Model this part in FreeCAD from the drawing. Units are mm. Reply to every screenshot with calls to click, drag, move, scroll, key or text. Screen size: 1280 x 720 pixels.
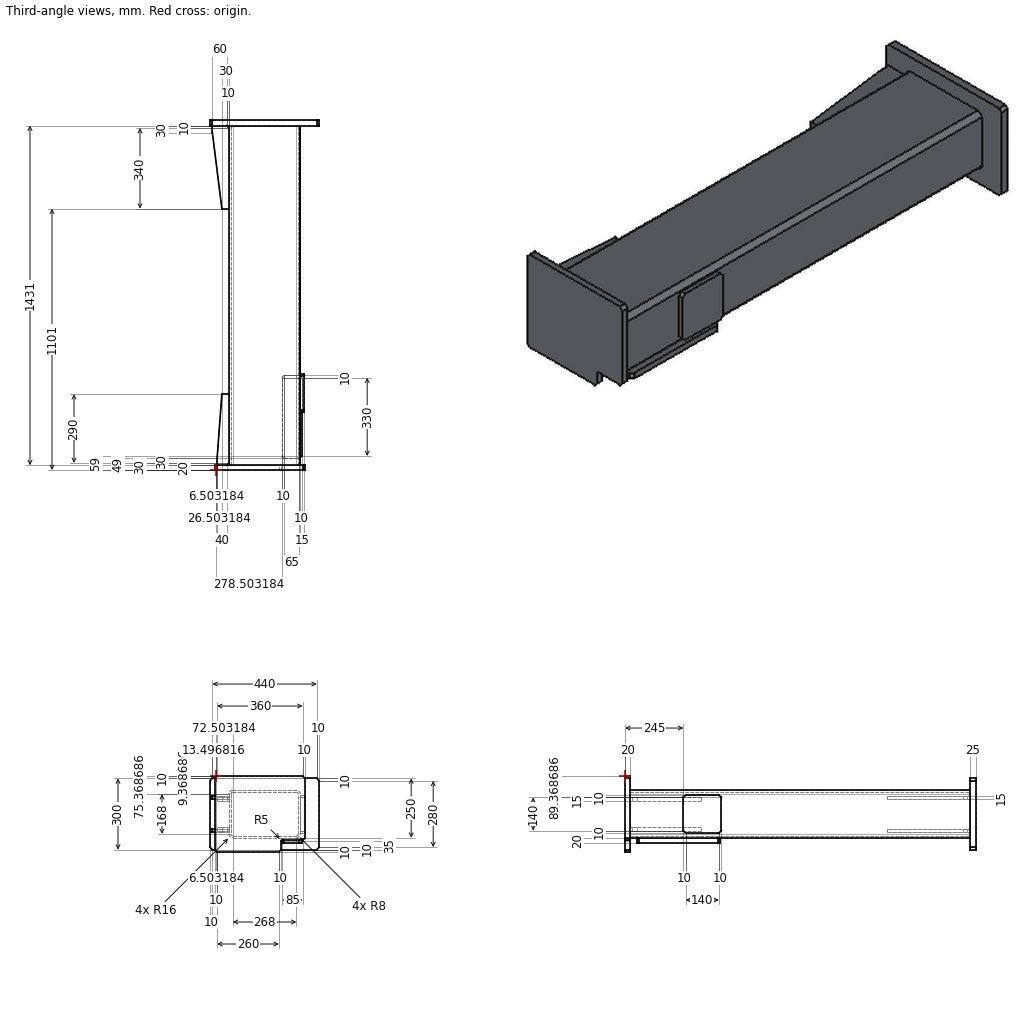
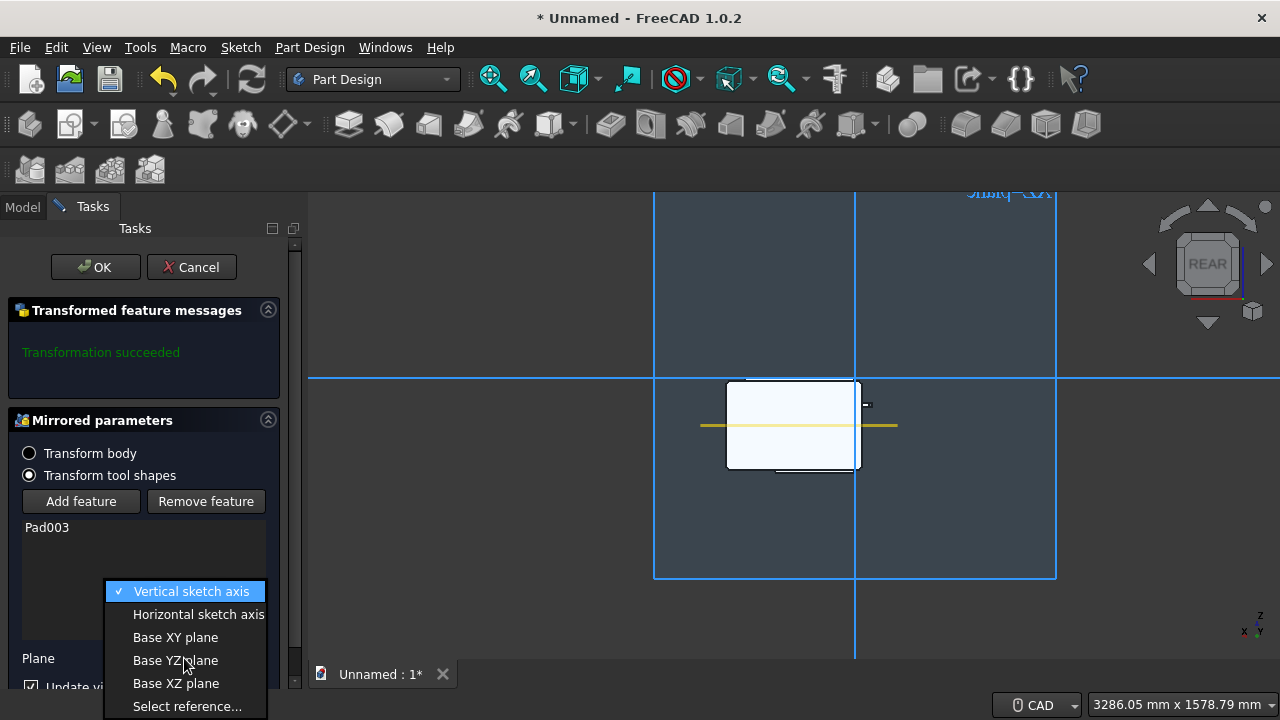
click(184, 706)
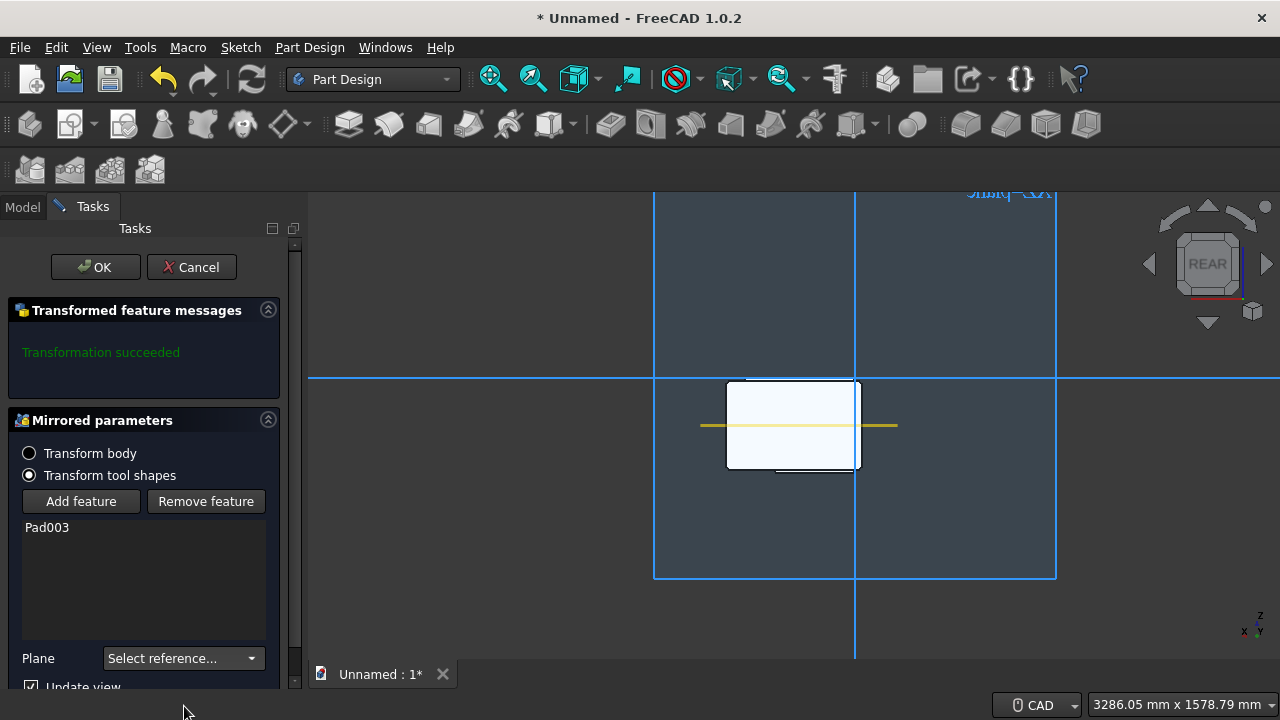
click(23, 206)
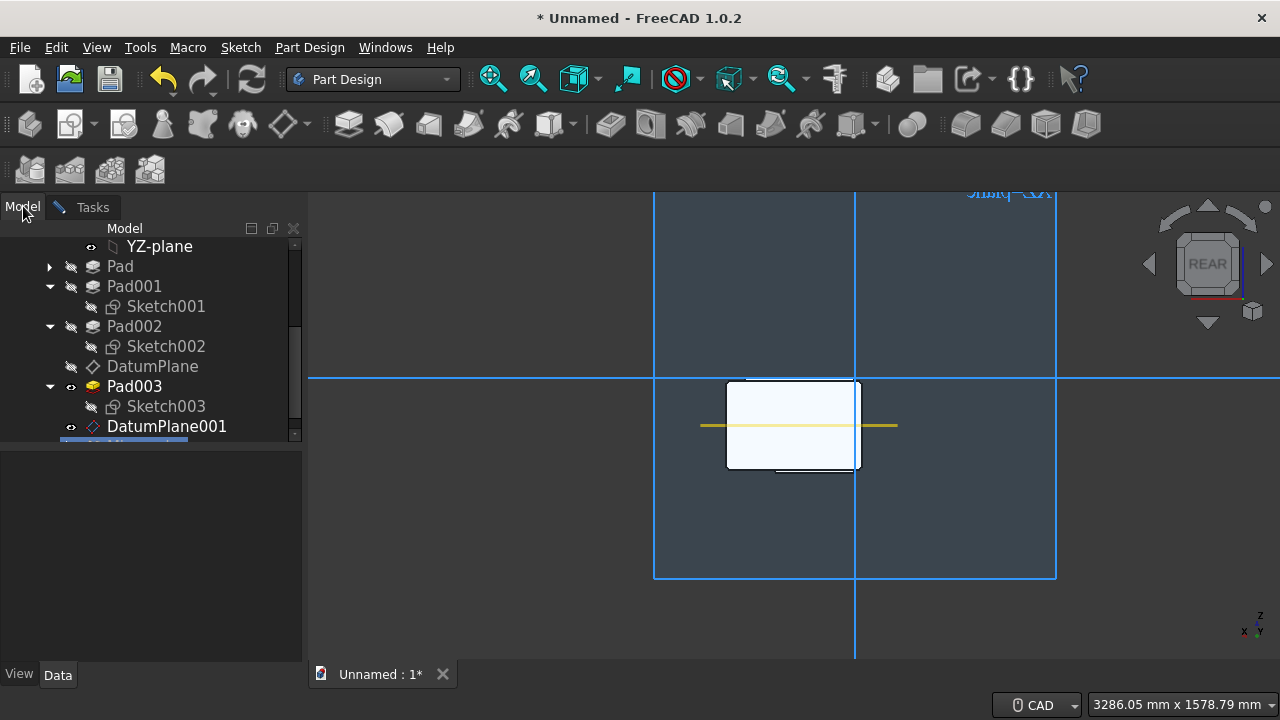
click(116, 427)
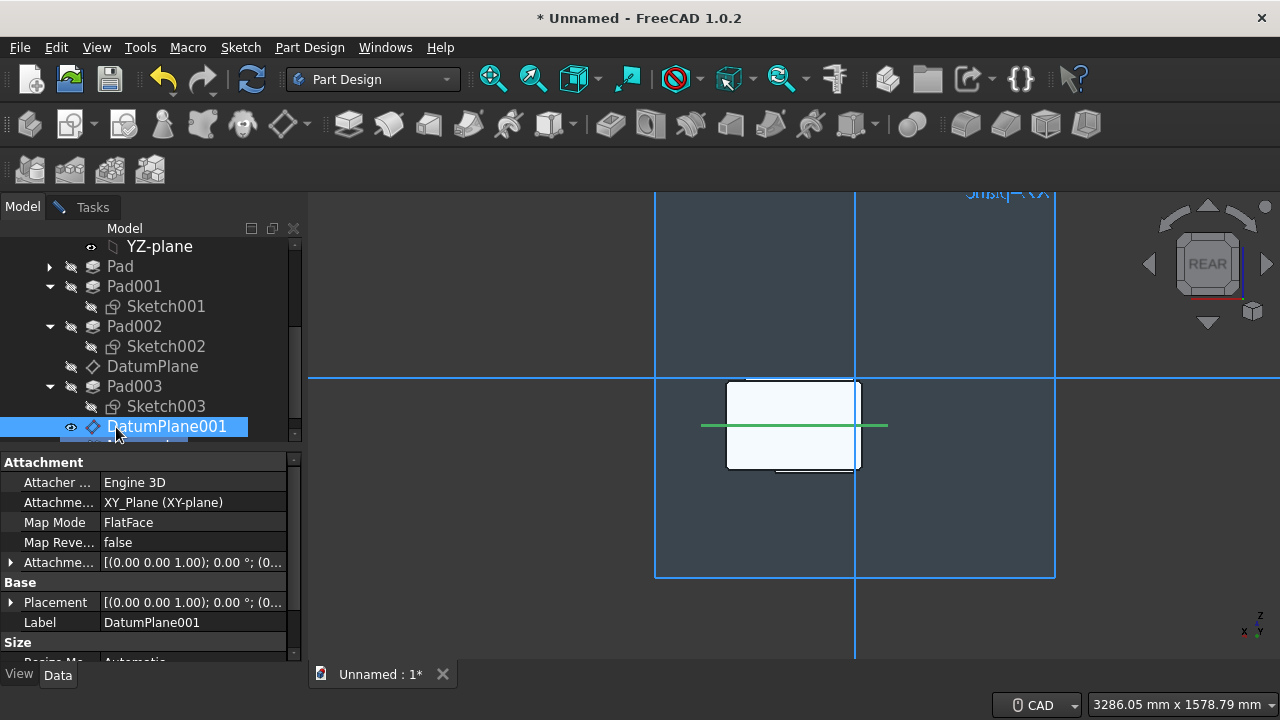
click(84, 206)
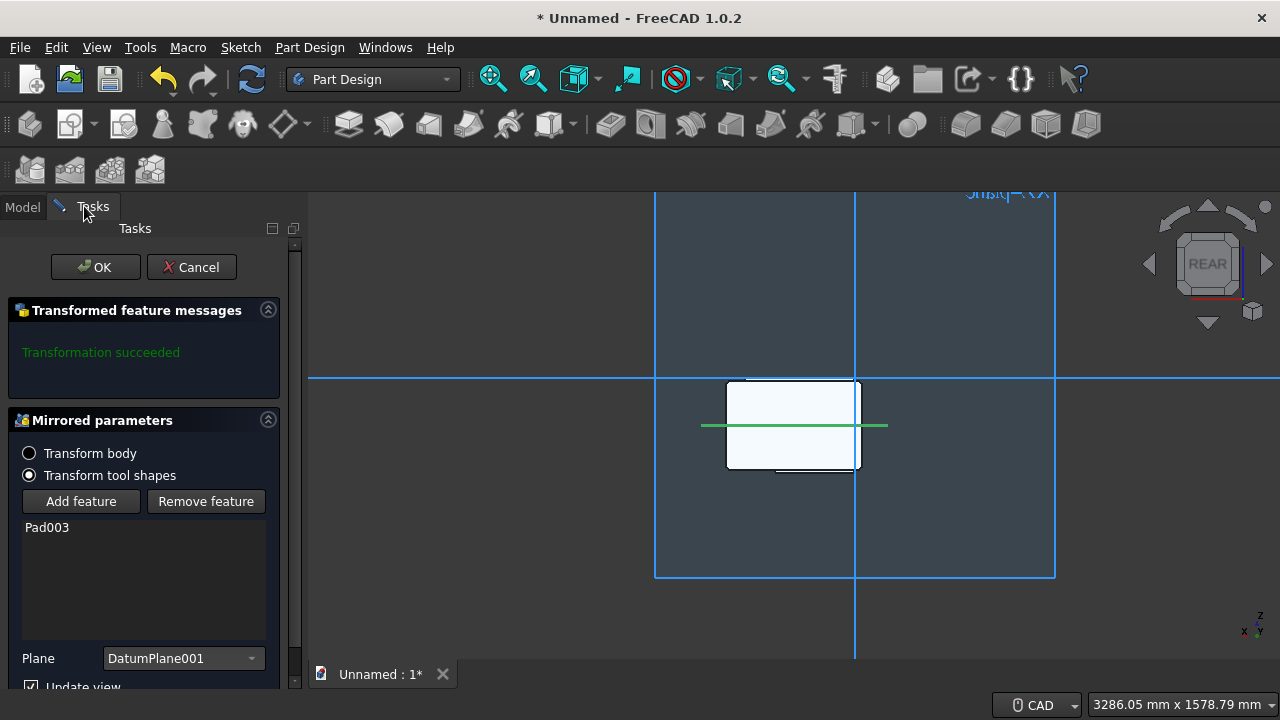
click(96, 267)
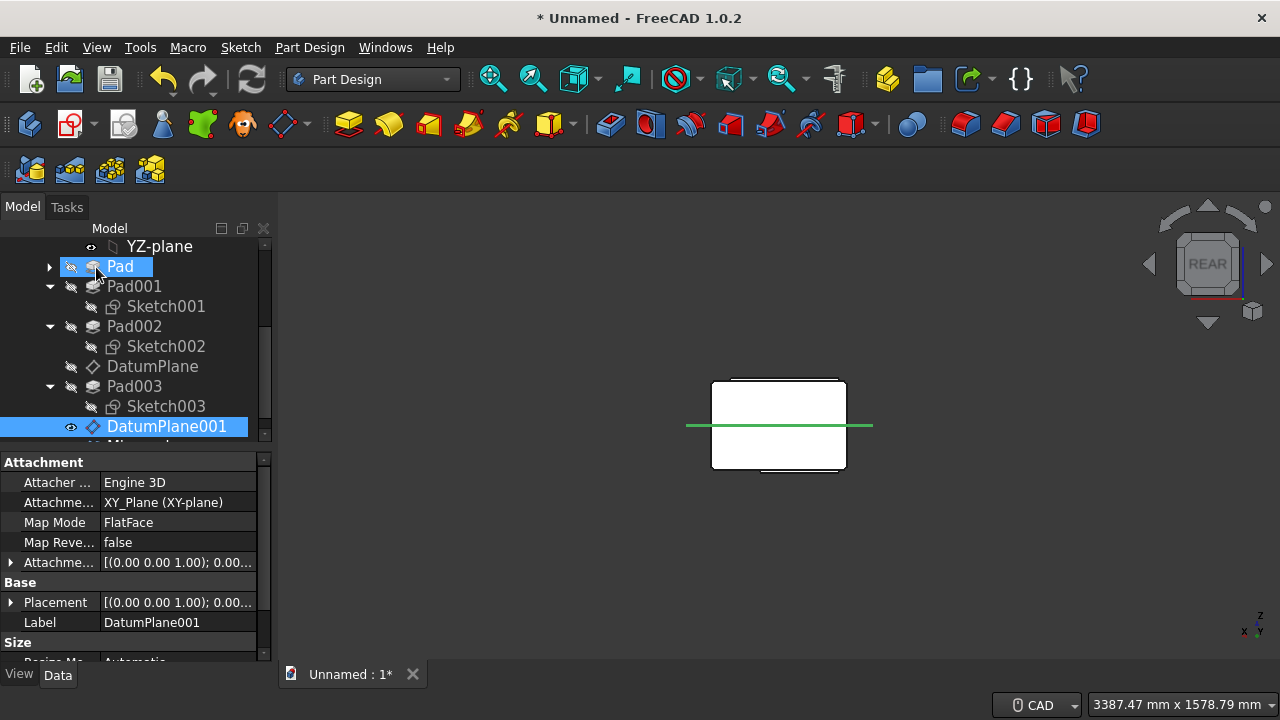
click(116, 427)
key(space)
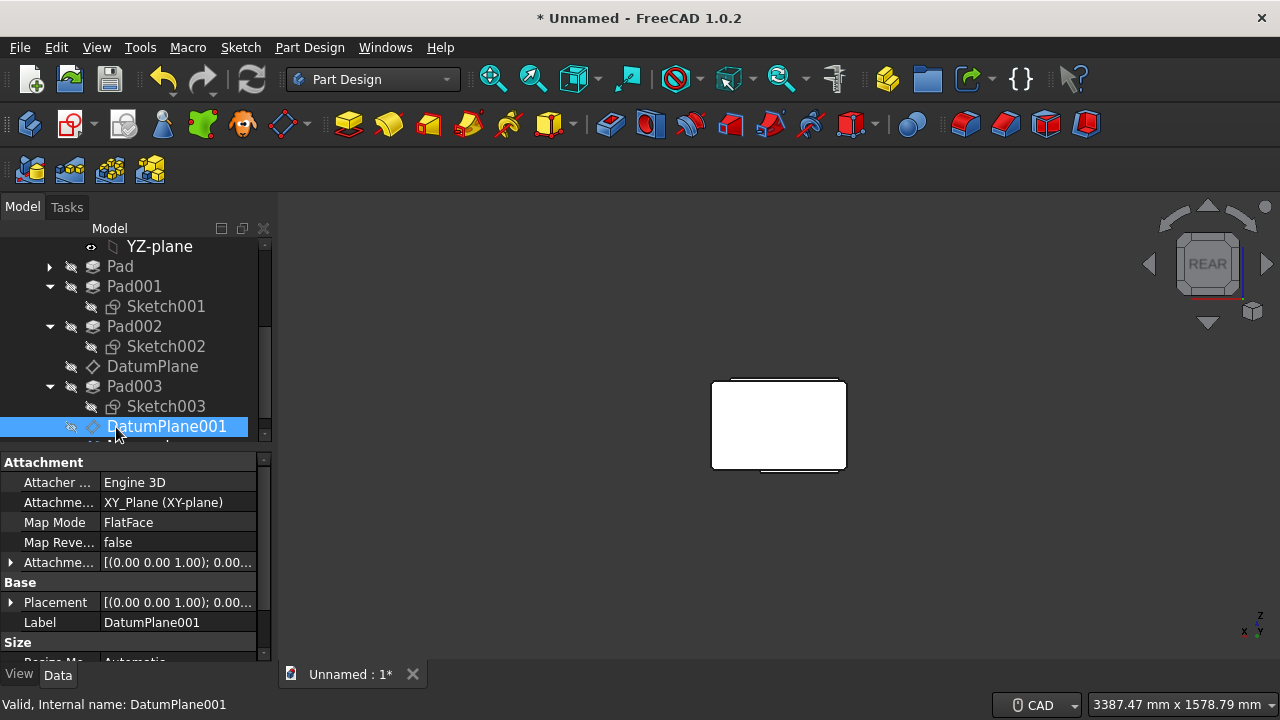
click(494, 80)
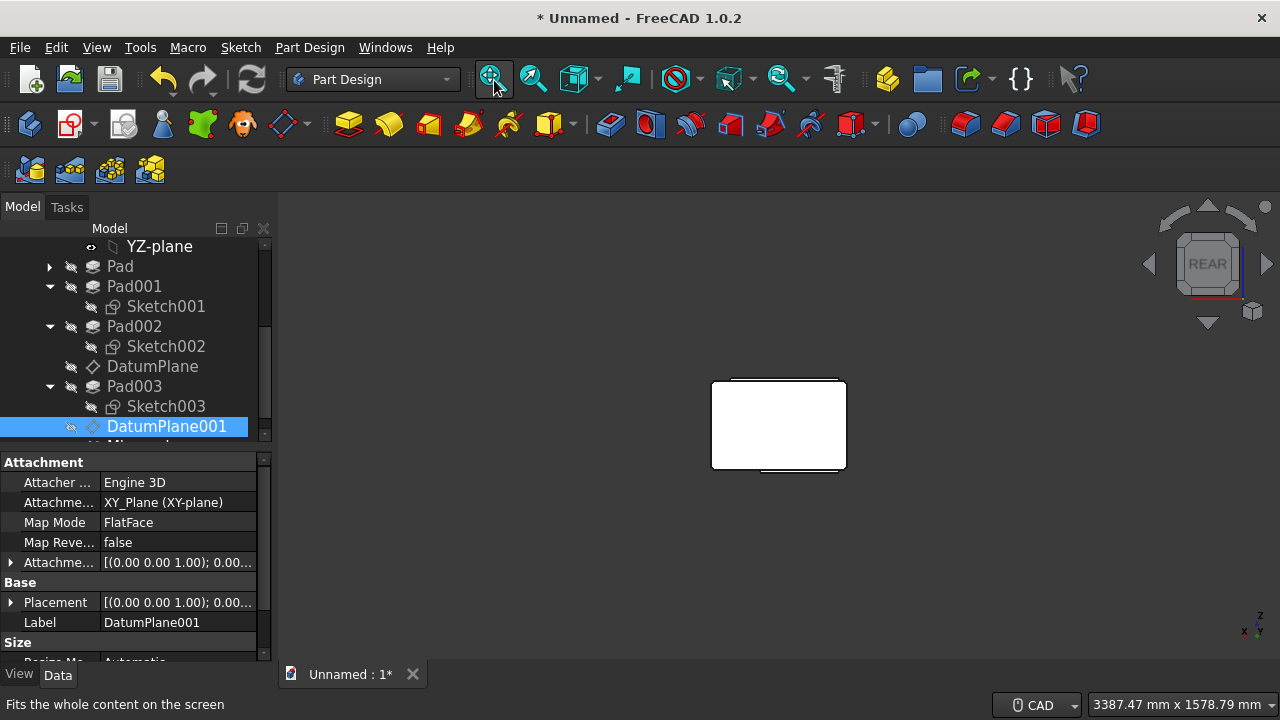
key(0)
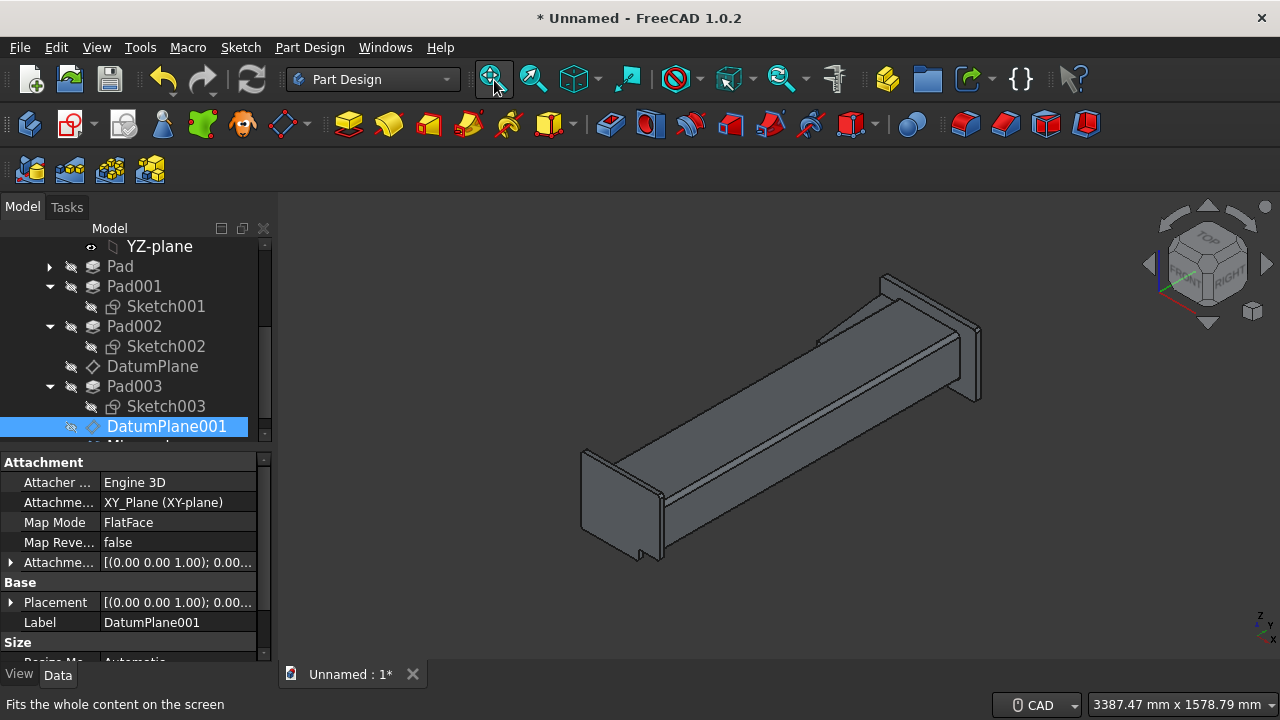
click(895, 394)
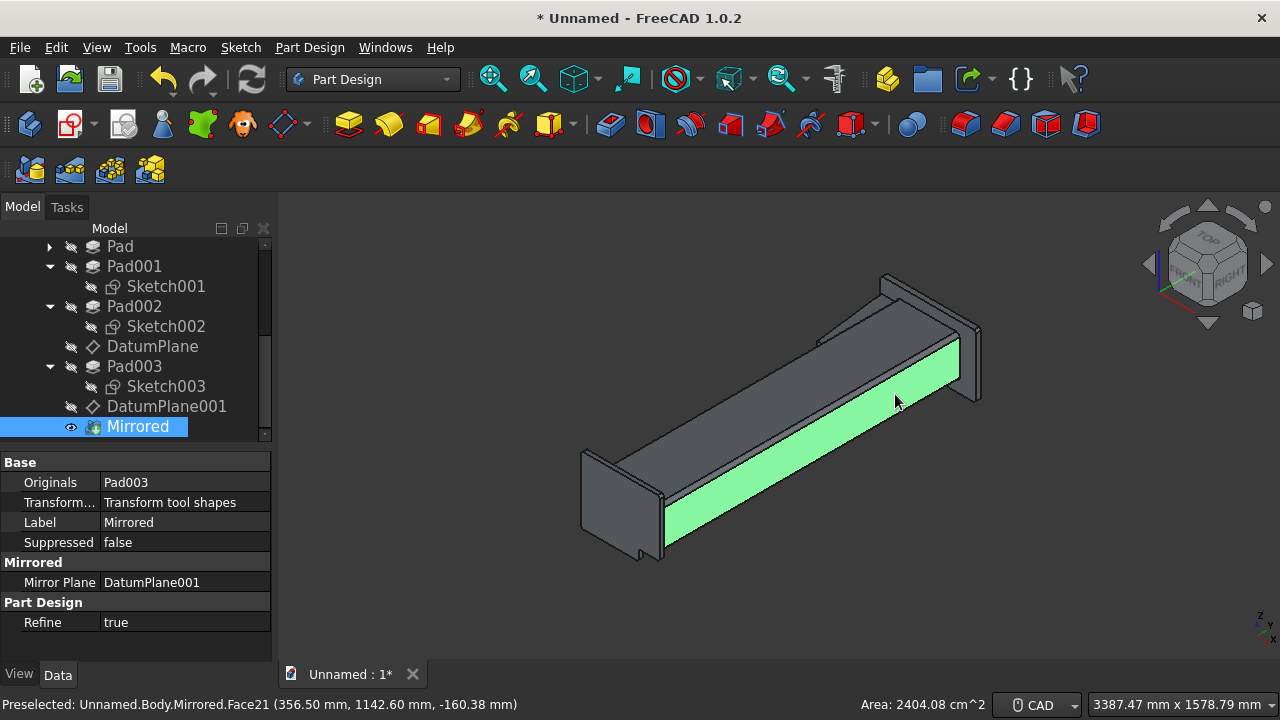
click(70, 124)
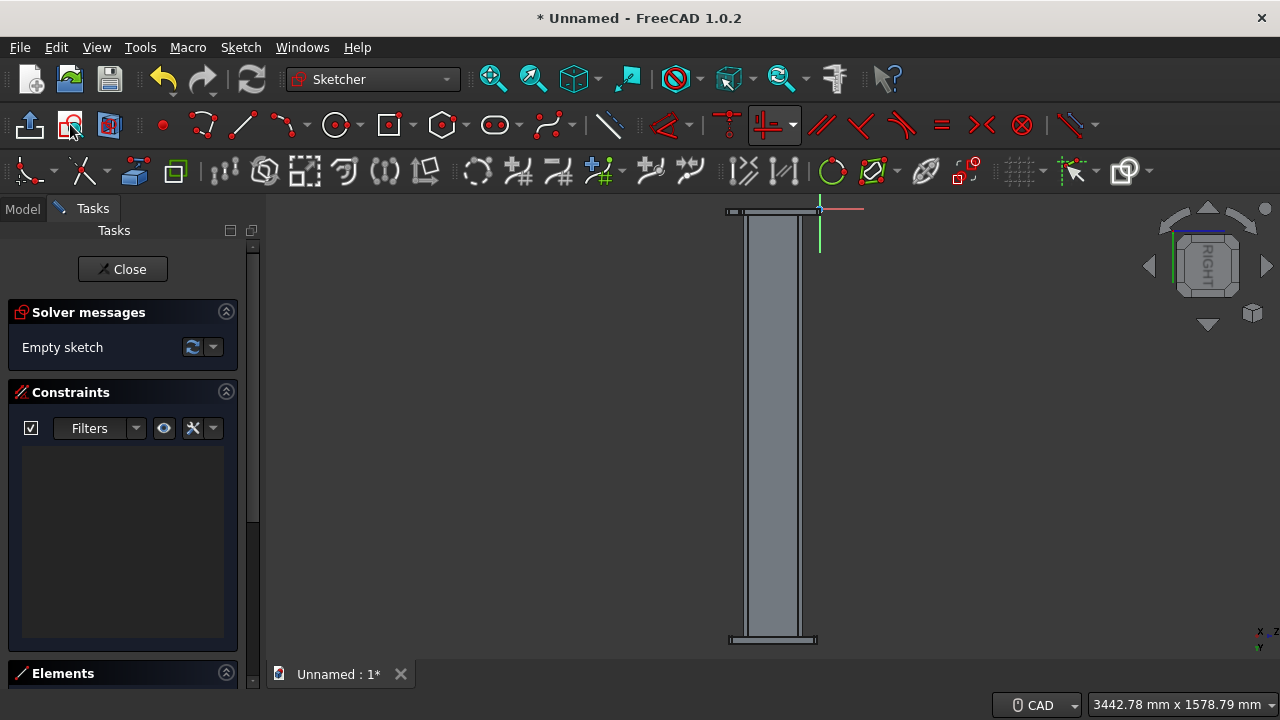
scroll(787, 281, up, 9)